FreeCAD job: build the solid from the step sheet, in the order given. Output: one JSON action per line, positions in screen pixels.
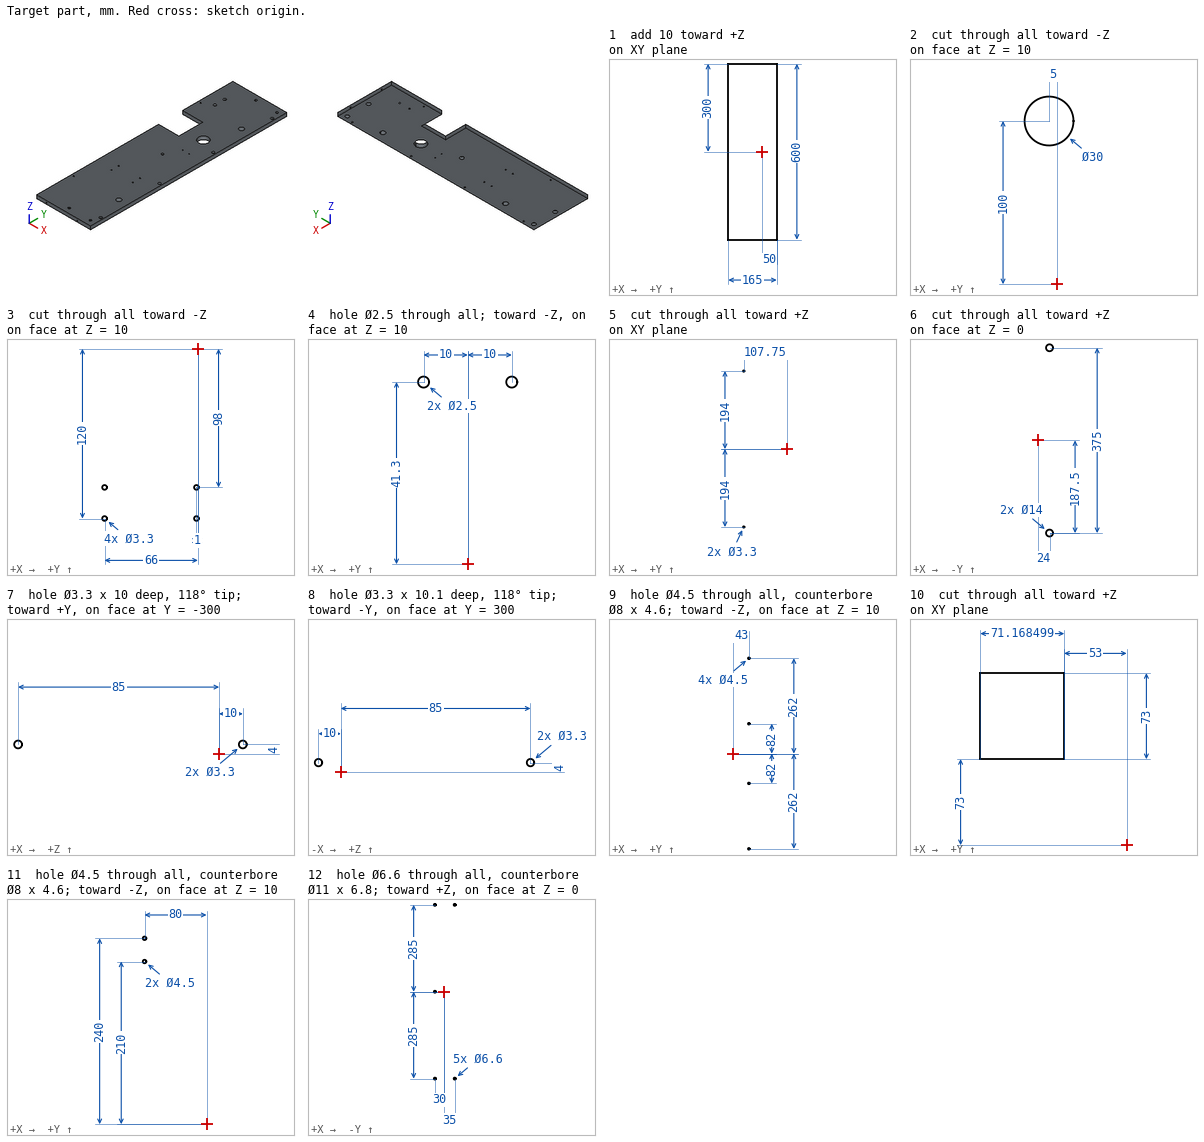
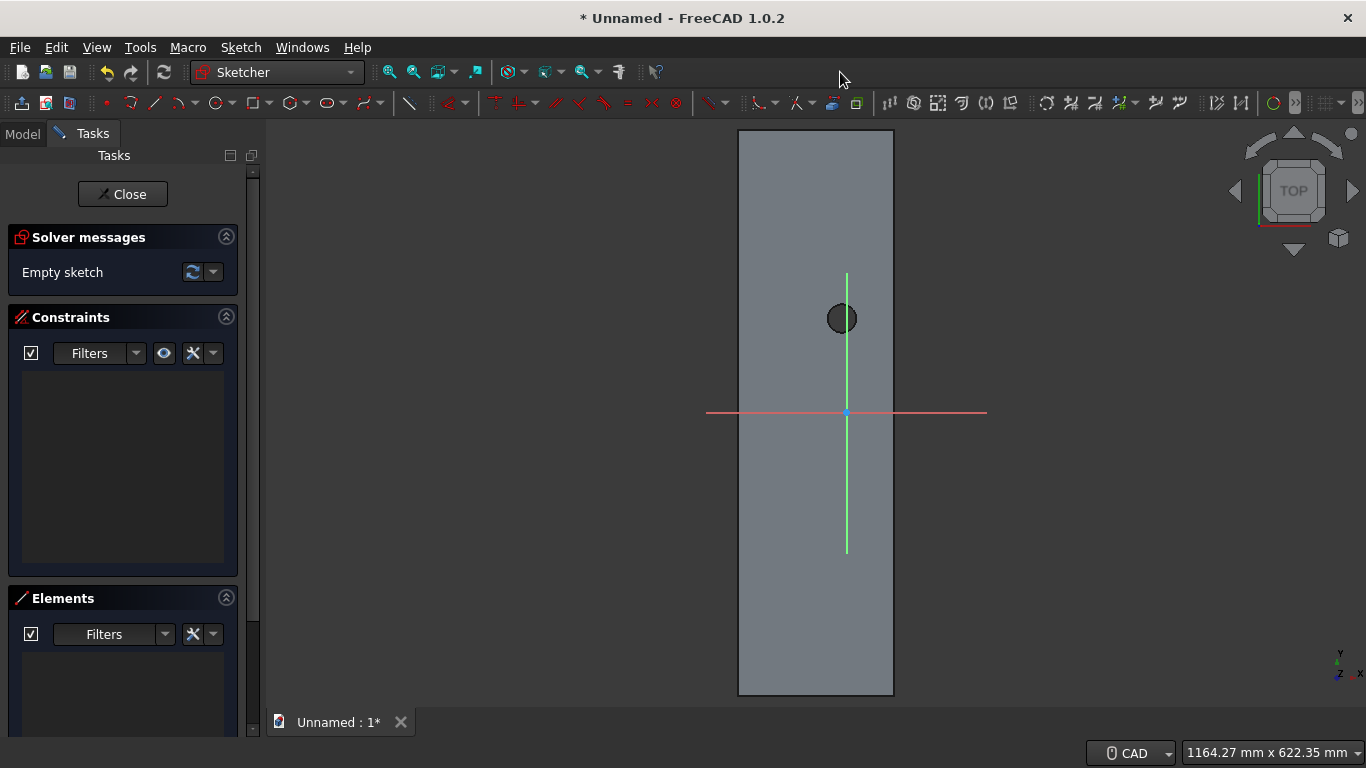
{"action": "scroll", "coordinate": [844, 495], "scroll_direction": "up", "scroll_amount": 6}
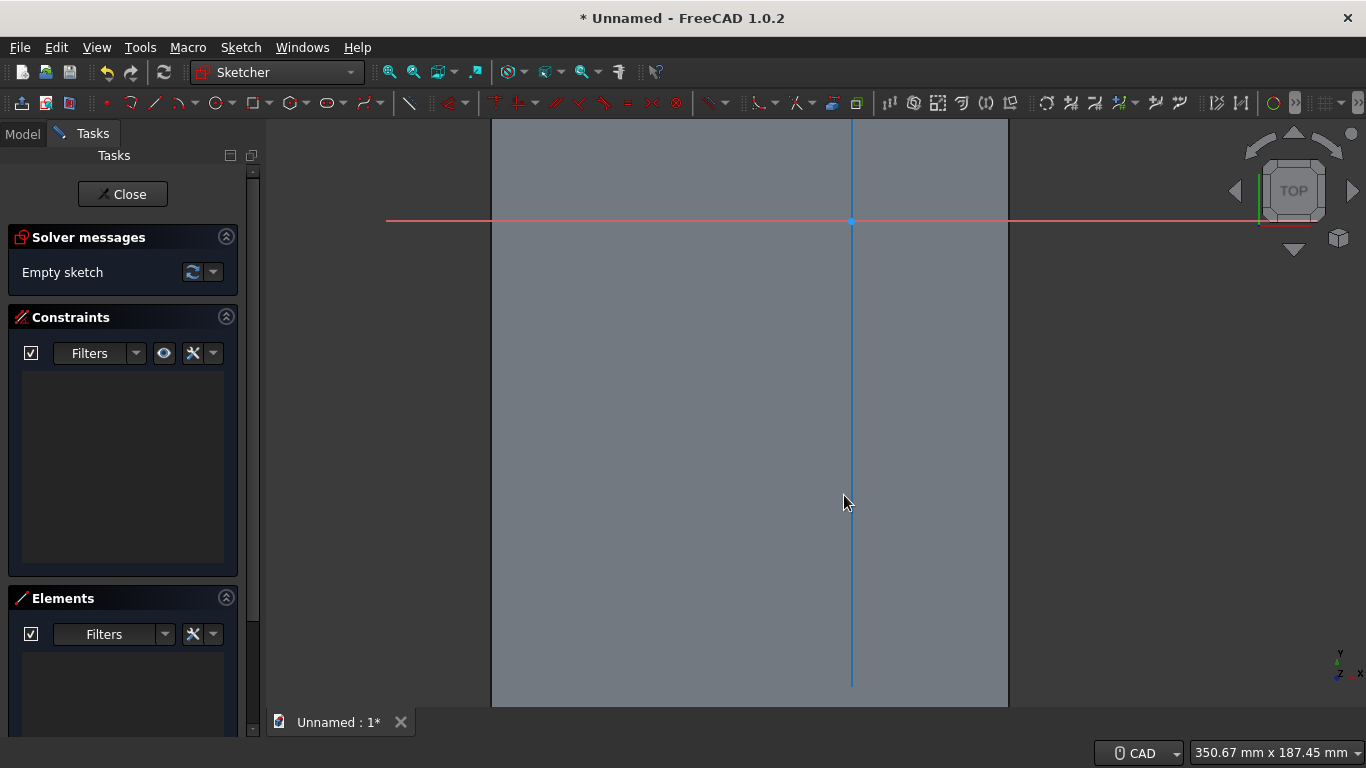
{"action": "left_click", "coordinate": [216, 104]}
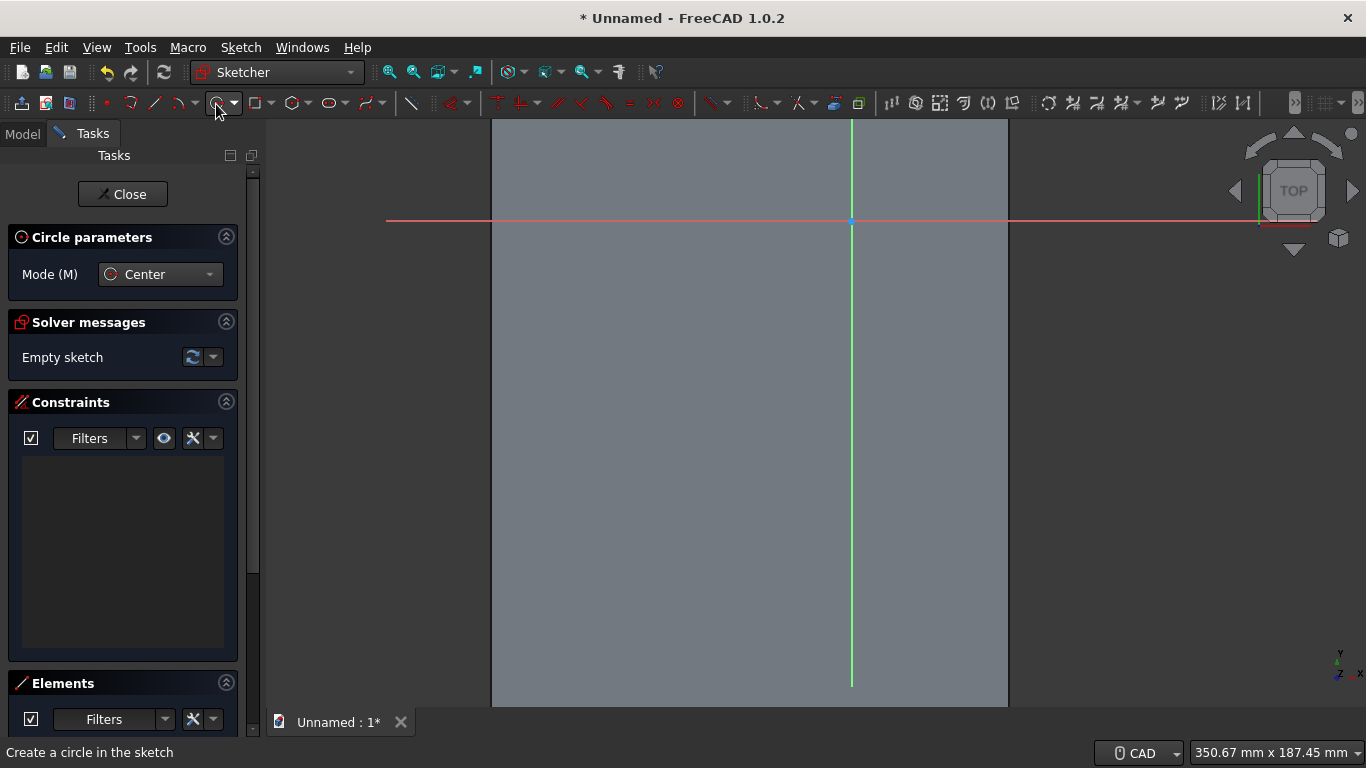
{"action": "scroll", "coordinate": [645, 598], "scroll_direction": "up", "scroll_amount": 8}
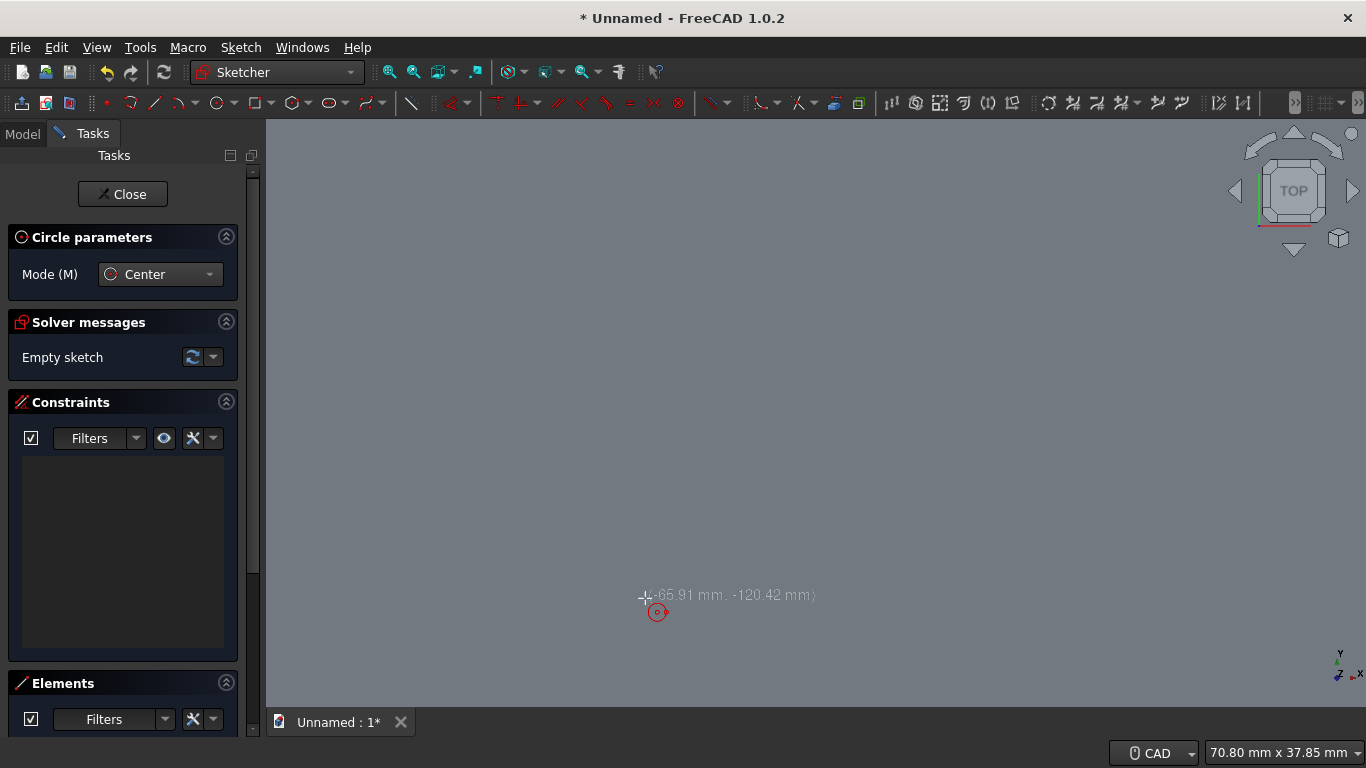
{"action": "scroll", "coordinate": [646, 600], "scroll_direction": "down", "scroll_amount": 8}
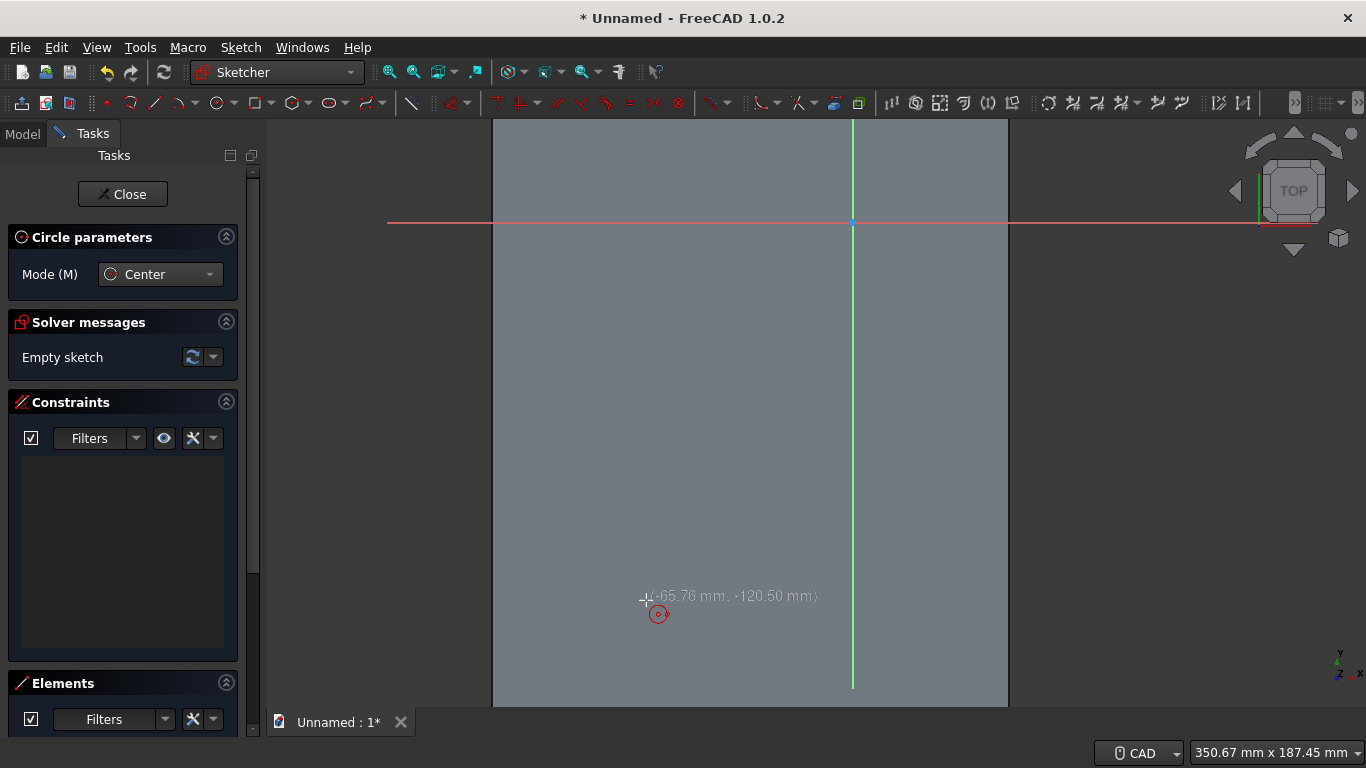
{"action": "left_click", "coordinate": [646, 599]}
{"action": "mouse_move", "coordinate": [649, 596]}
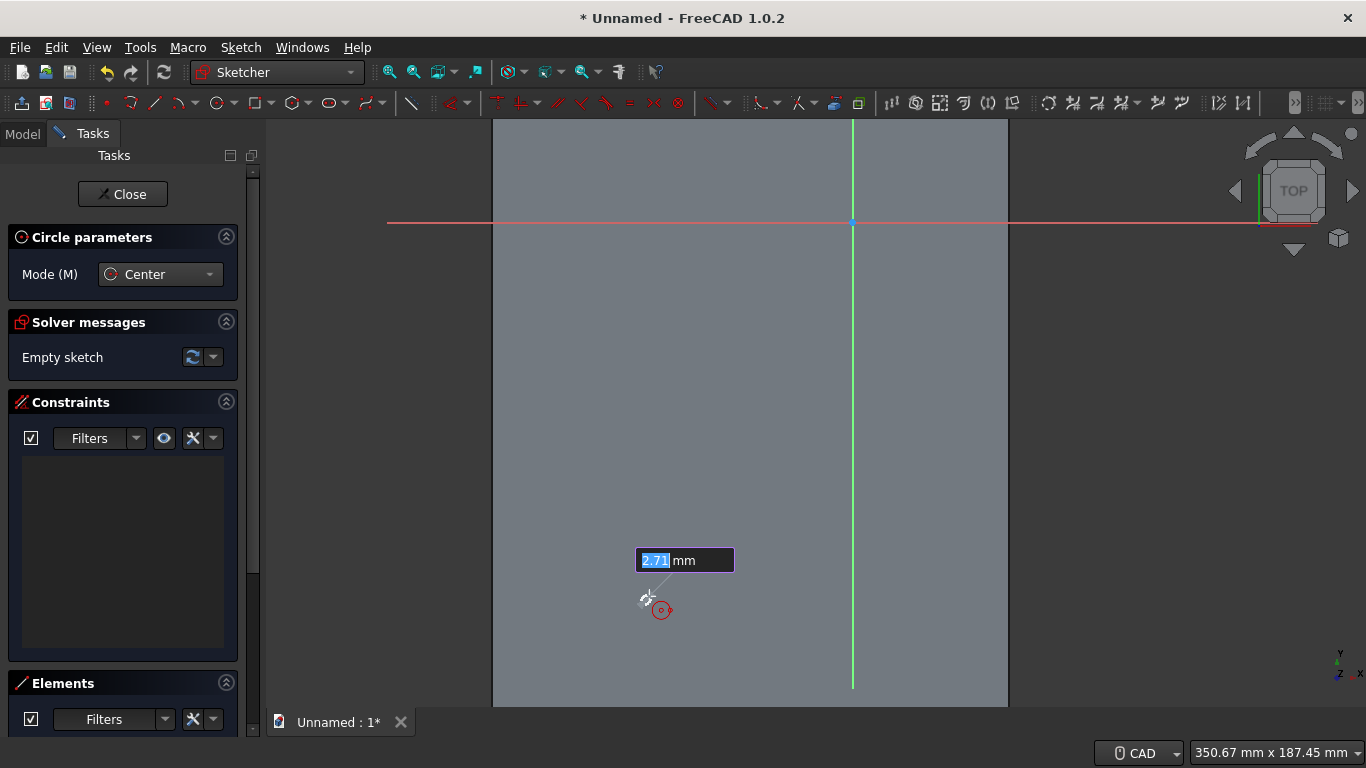
{"action": "type", "text": "3.3"}
{"action": "key", "text": "Return"}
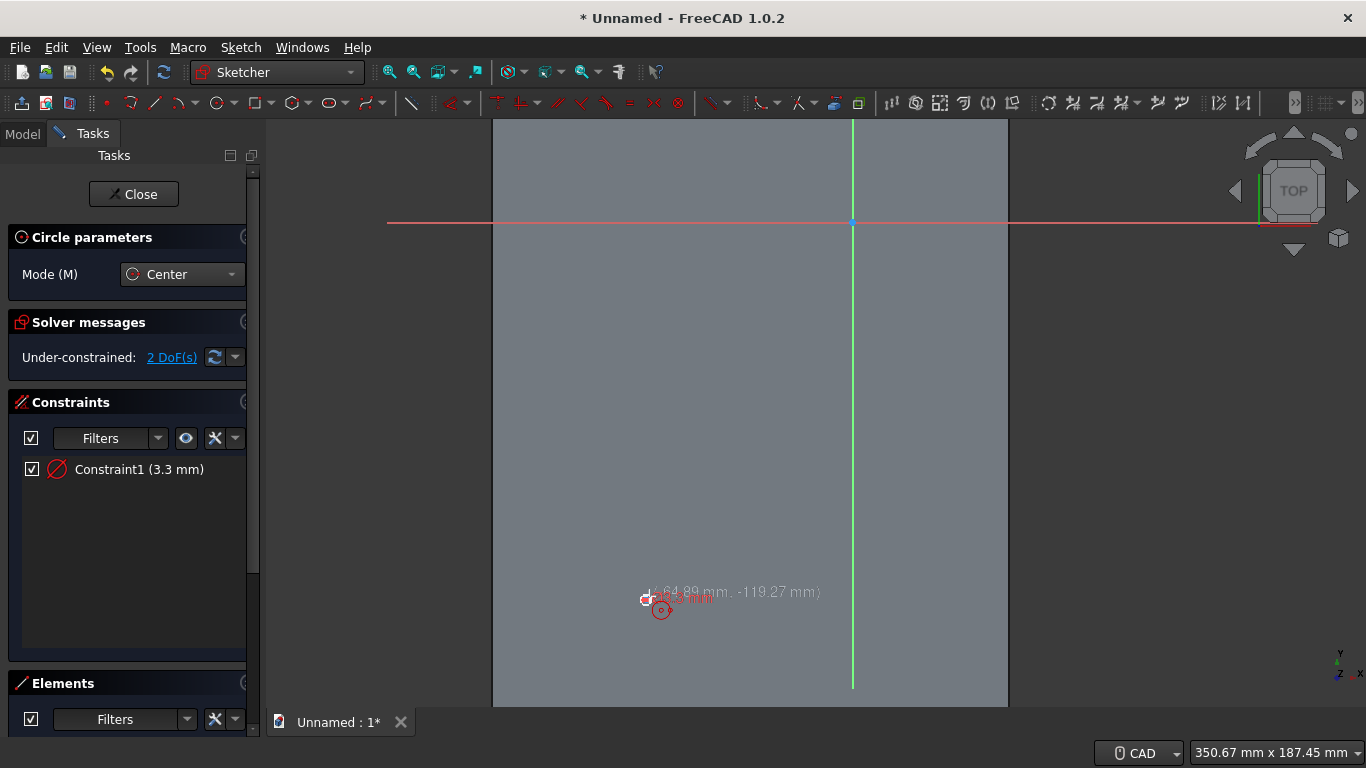
{"action": "scroll", "coordinate": [849, 530], "scroll_direction": "up", "scroll_amount": 9}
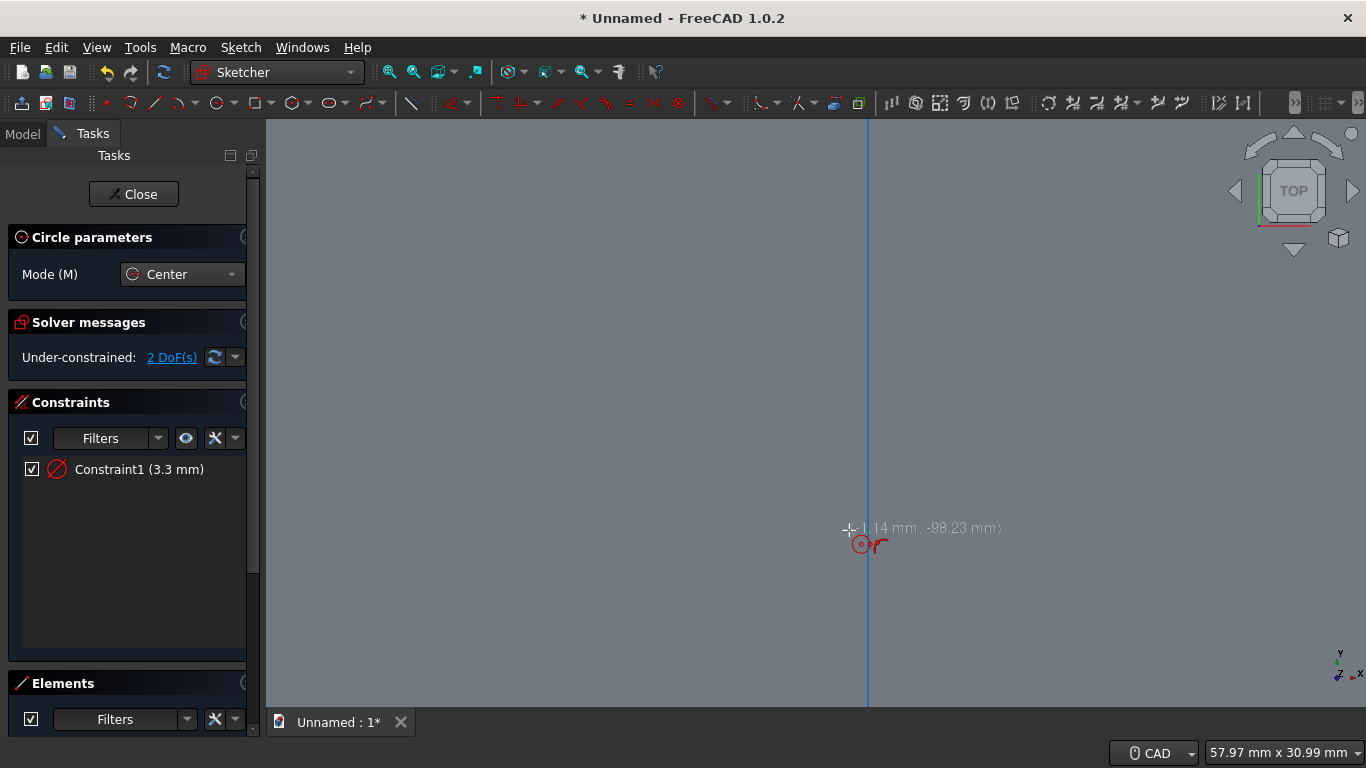
{"action": "left_click", "coordinate": [849, 528]}
{"action": "mouse_move", "coordinate": [827, 506]}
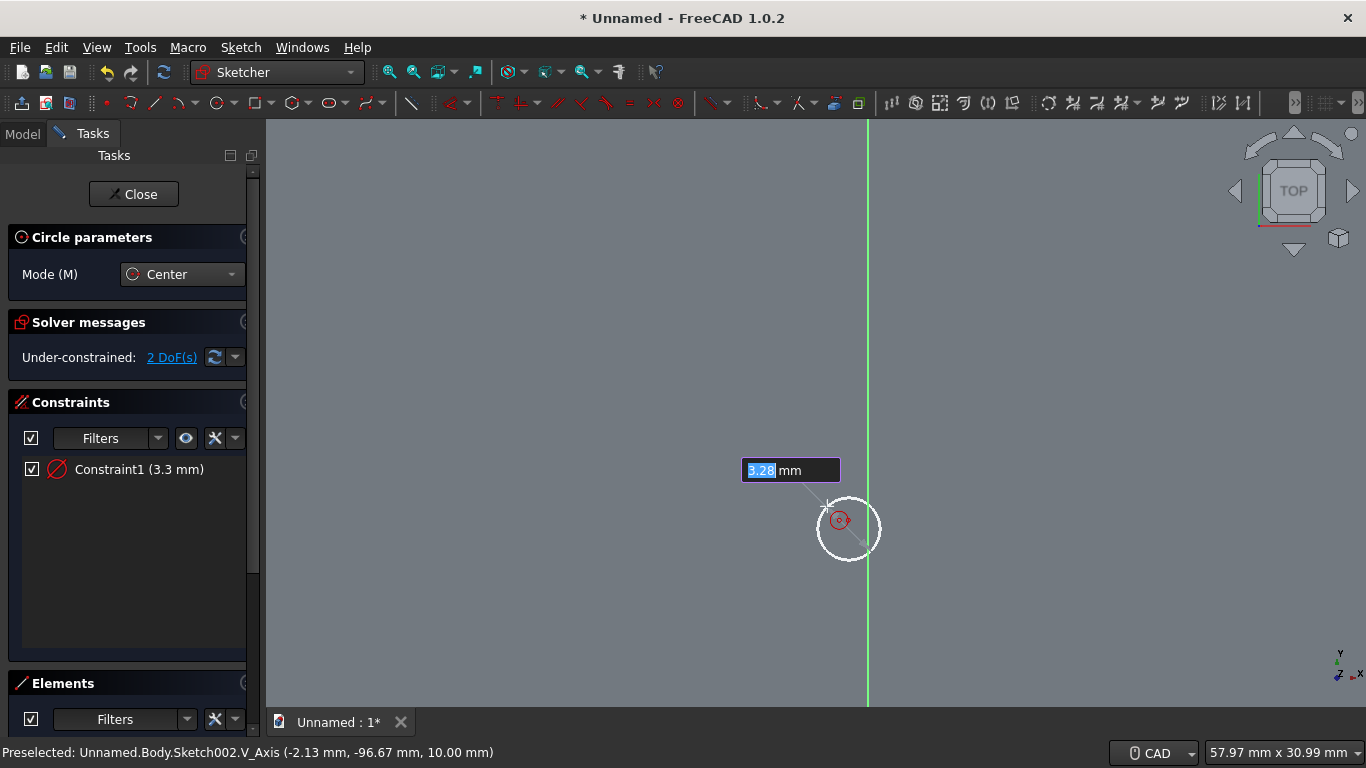
{"action": "type", "text": "3.3"}
{"action": "key", "text": "Return"}